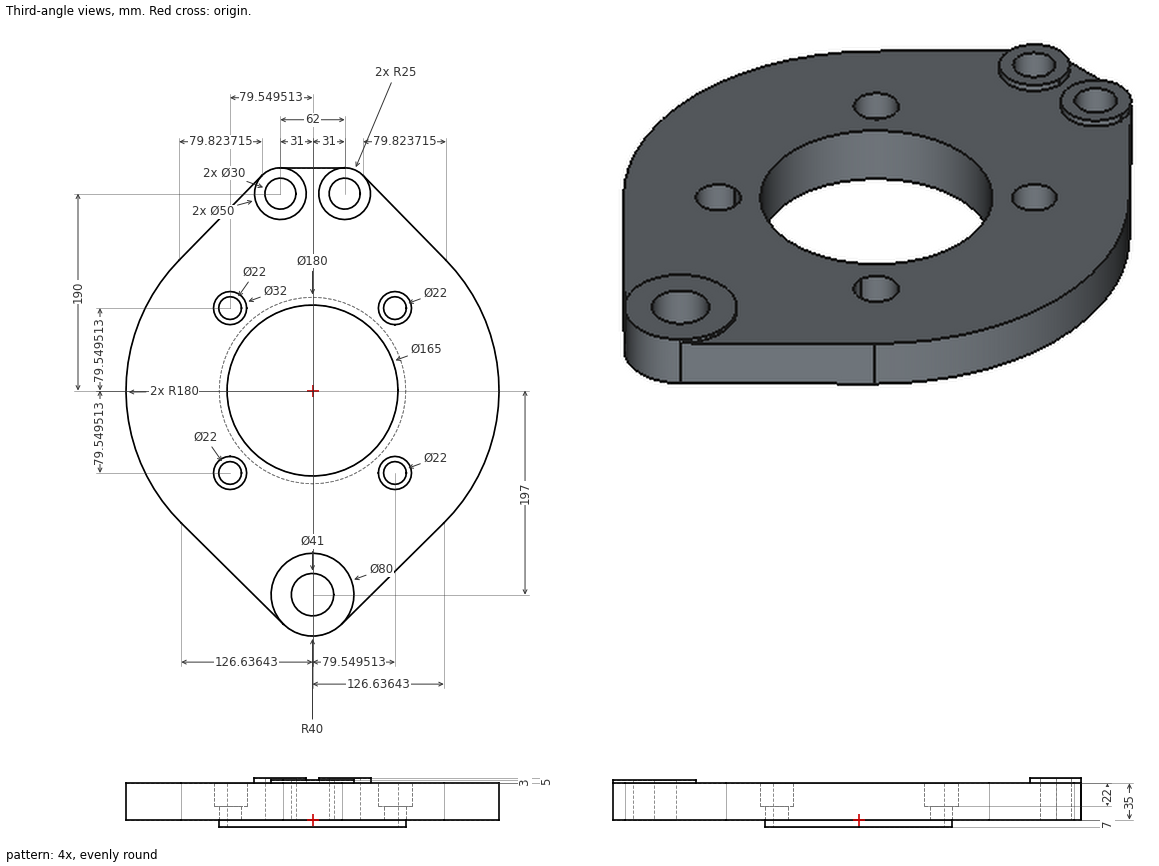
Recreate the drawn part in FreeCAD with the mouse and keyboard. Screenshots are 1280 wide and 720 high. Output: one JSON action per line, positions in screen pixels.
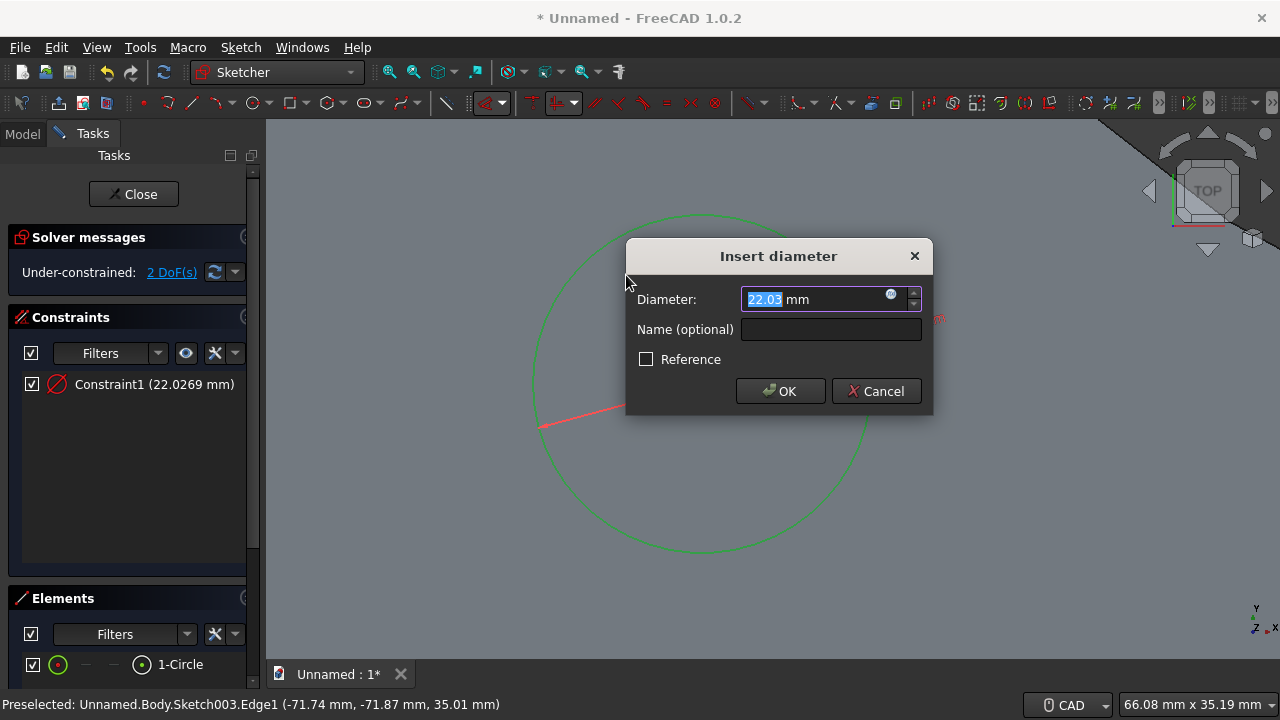
{"action": "type", "text": "22"}
{"action": "key", "text": "Return"}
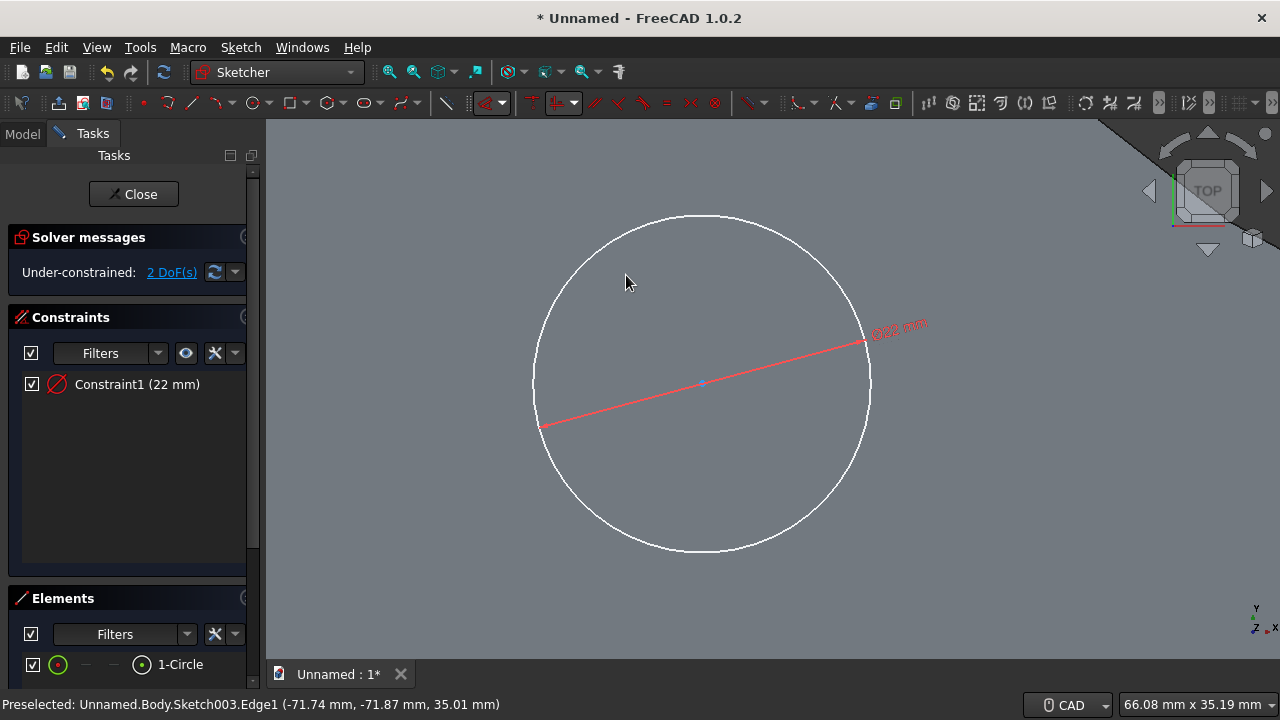
{"action": "left_click", "coordinate": [702, 384]}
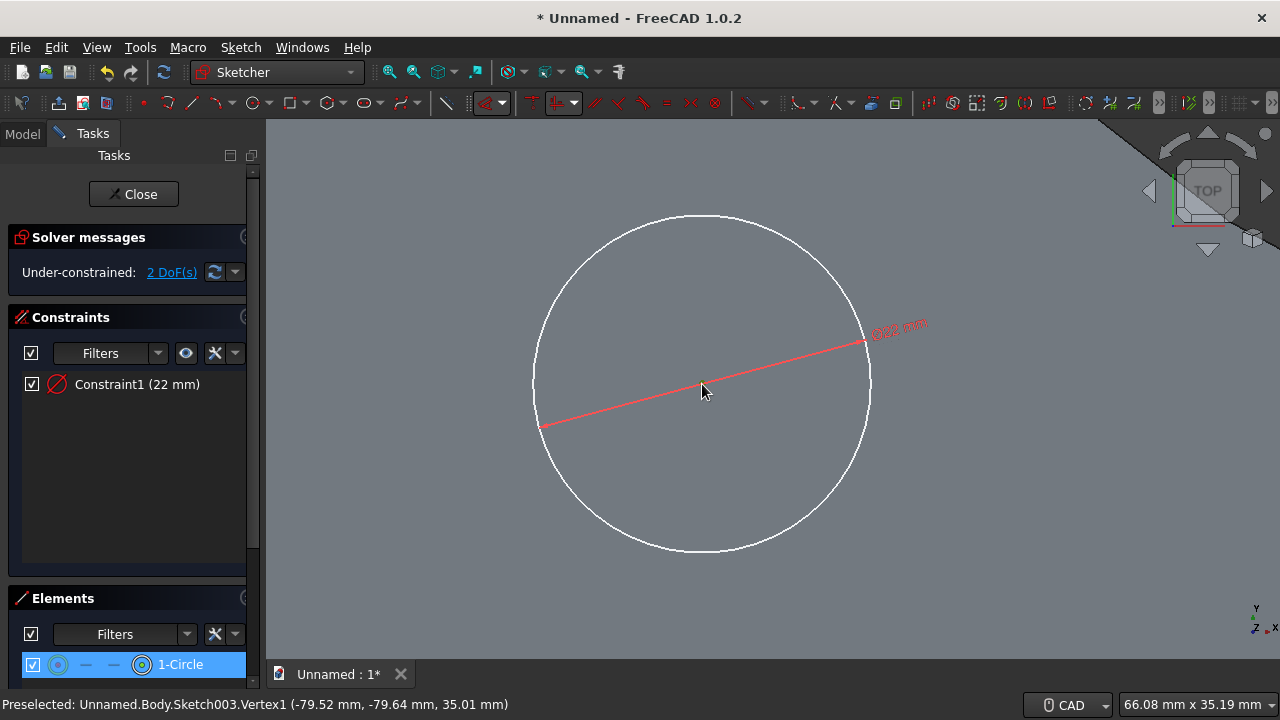
{"action": "key", "text": "l"}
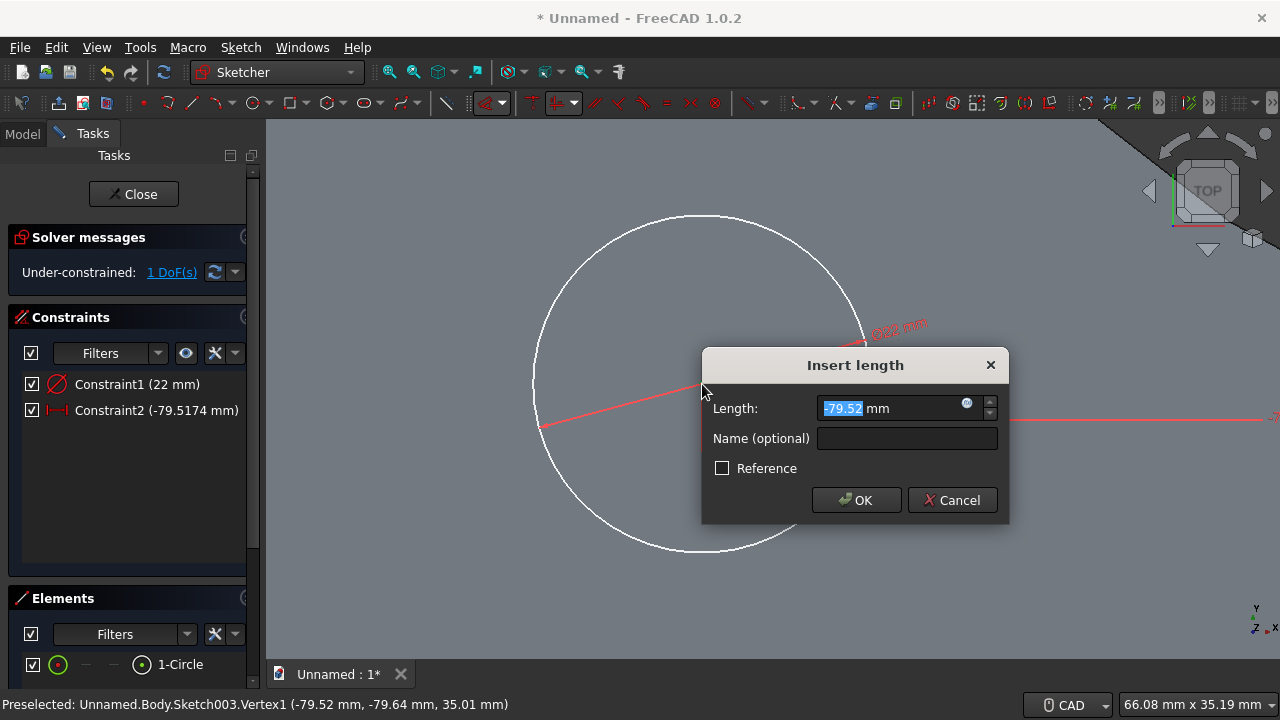
{"action": "type", "text": "-79.549513"}
{"action": "key", "text": "Return"}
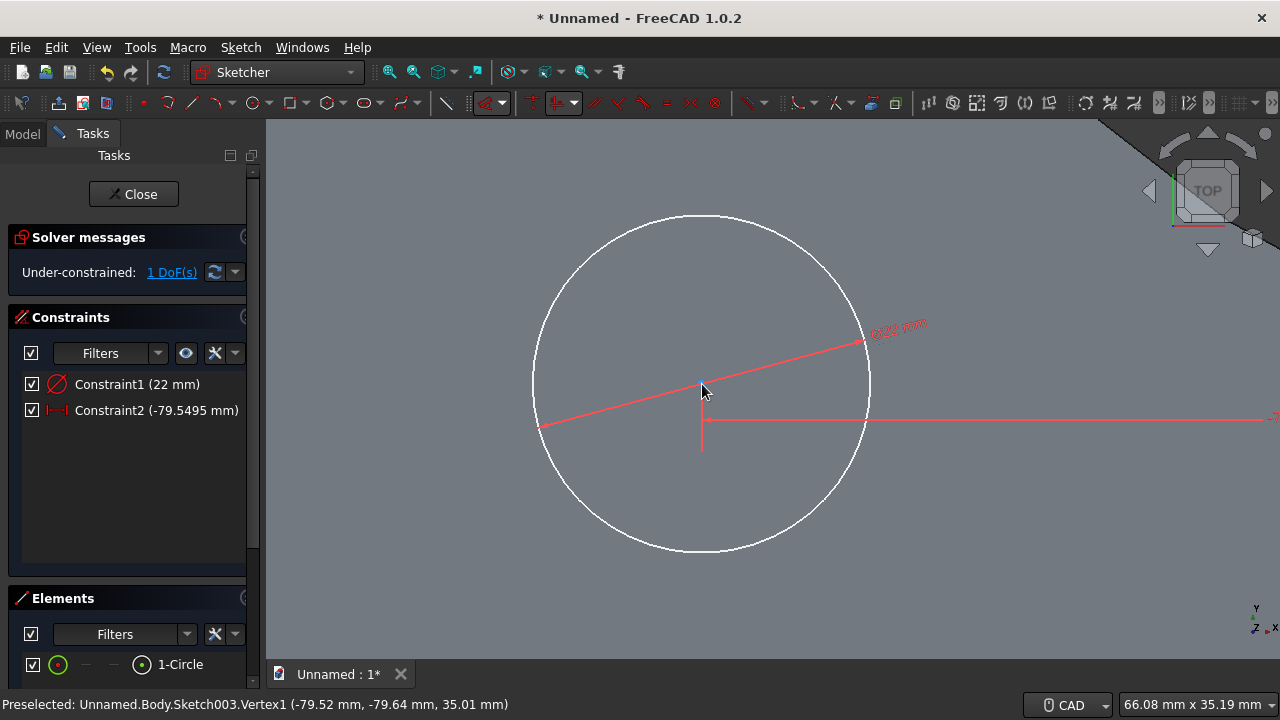
{"action": "left_click", "coordinate": [702, 384]}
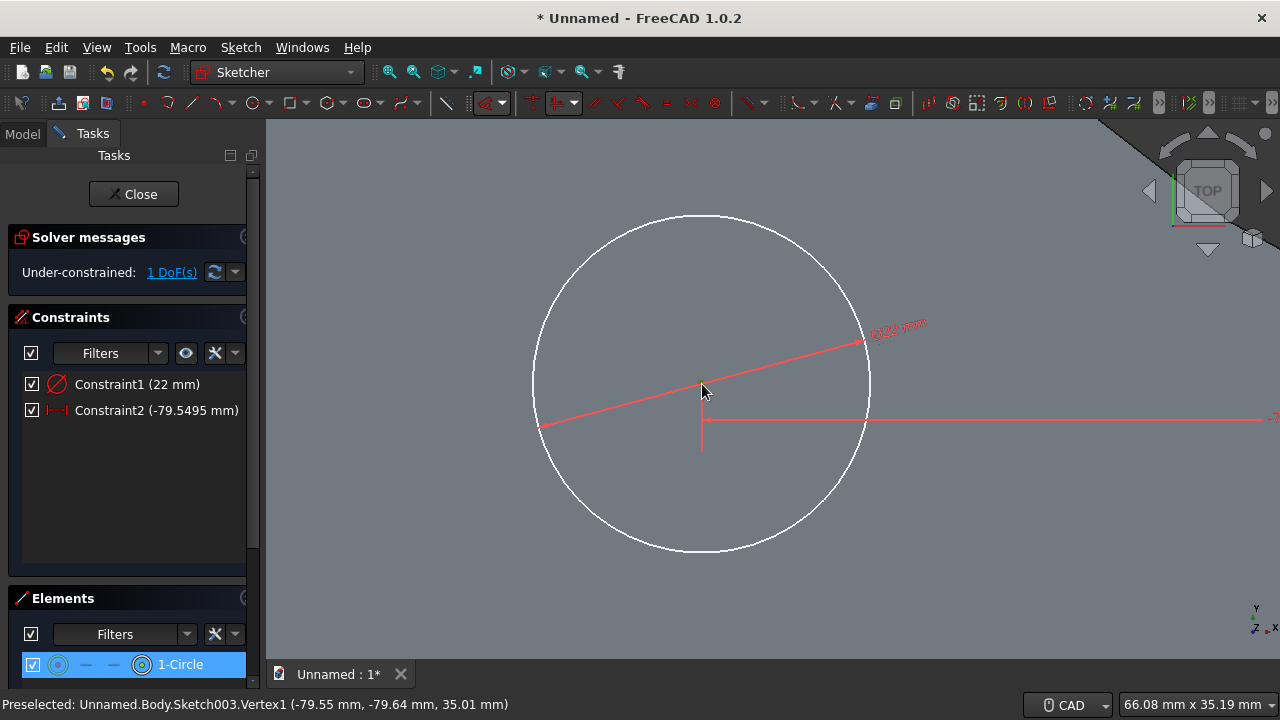
{"action": "left_click", "coordinate": [504, 104]}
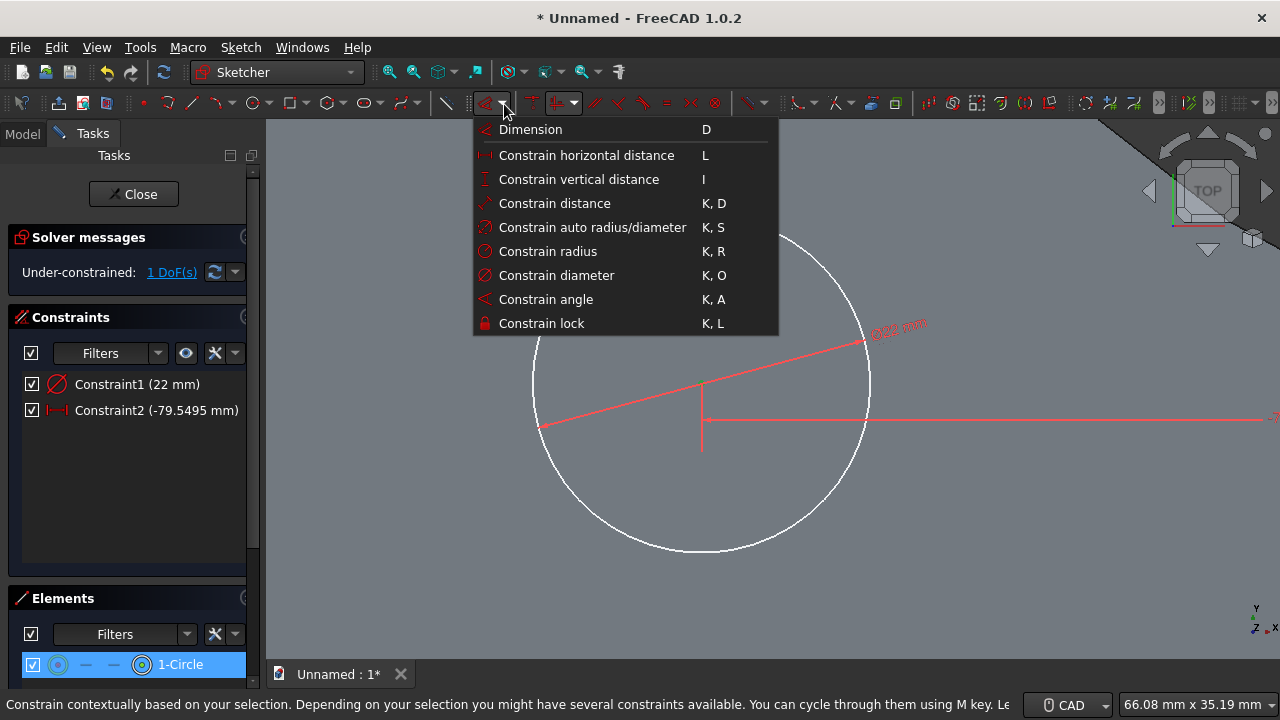
{"action": "left_click", "coordinate": [626, 179]}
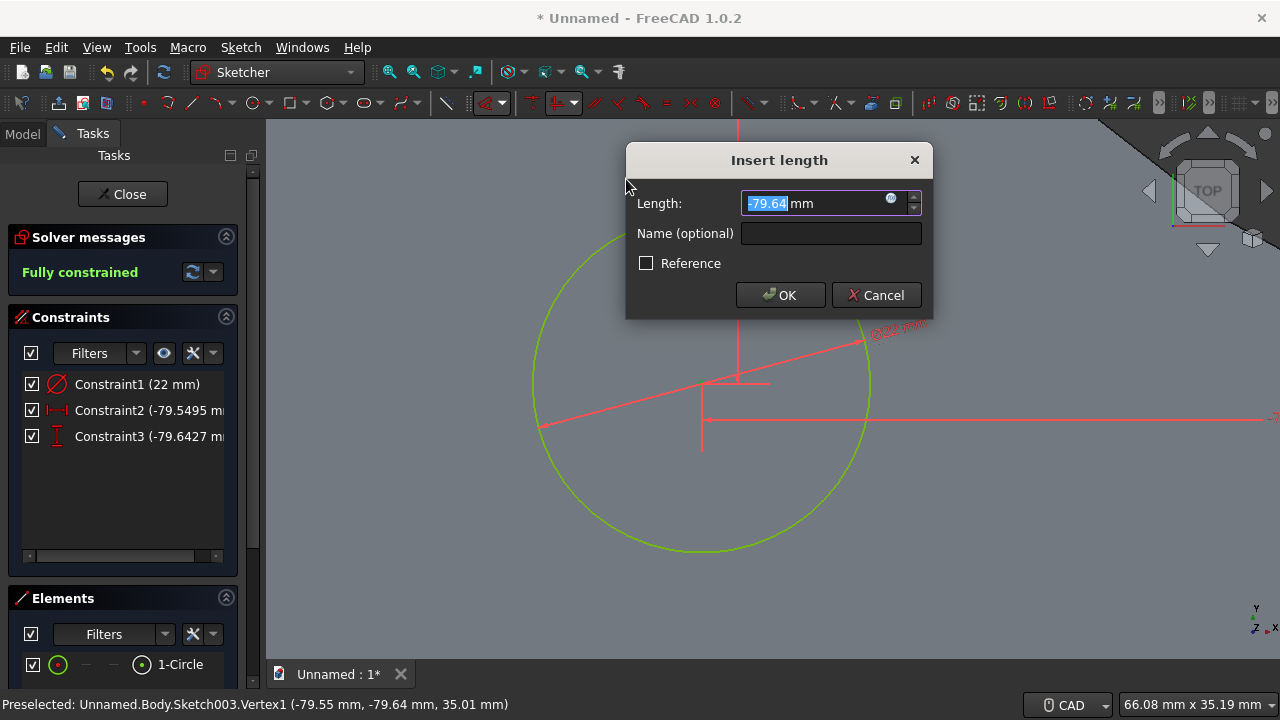
{"action": "type", "text": "-79.549513"}
{"action": "key", "text": "Return"}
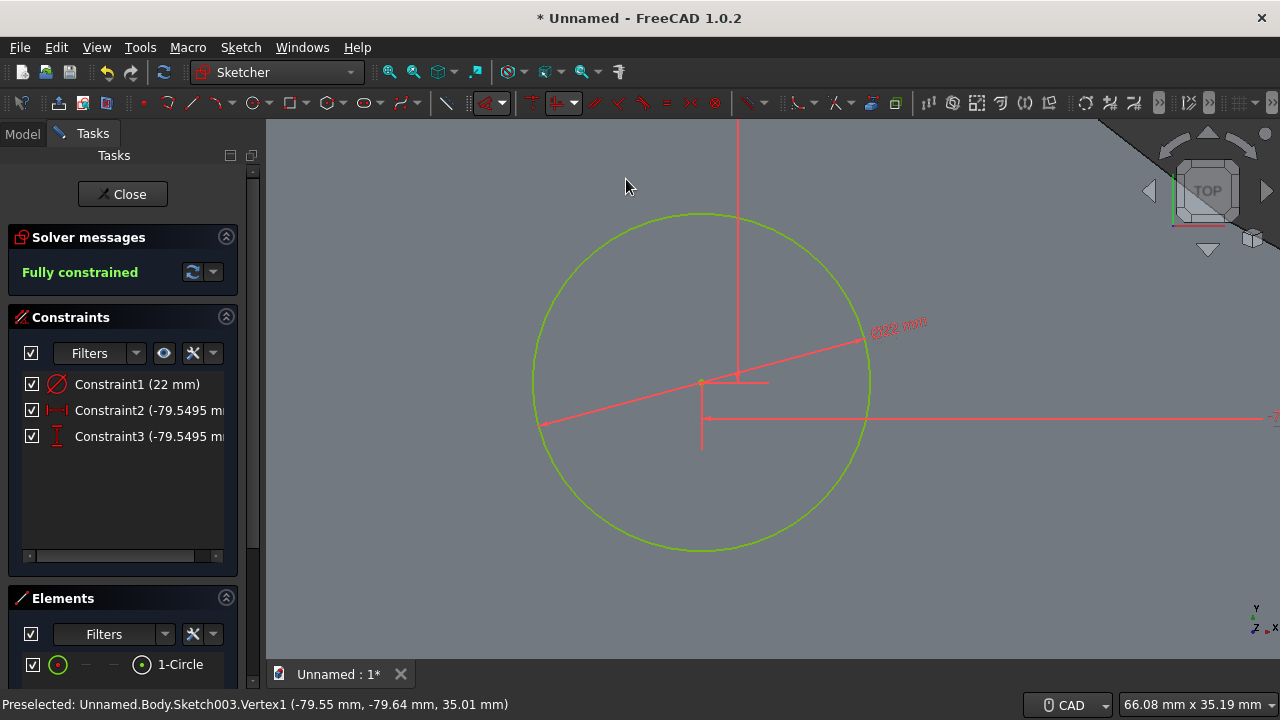
{"action": "left_click", "coordinate": [123, 194]}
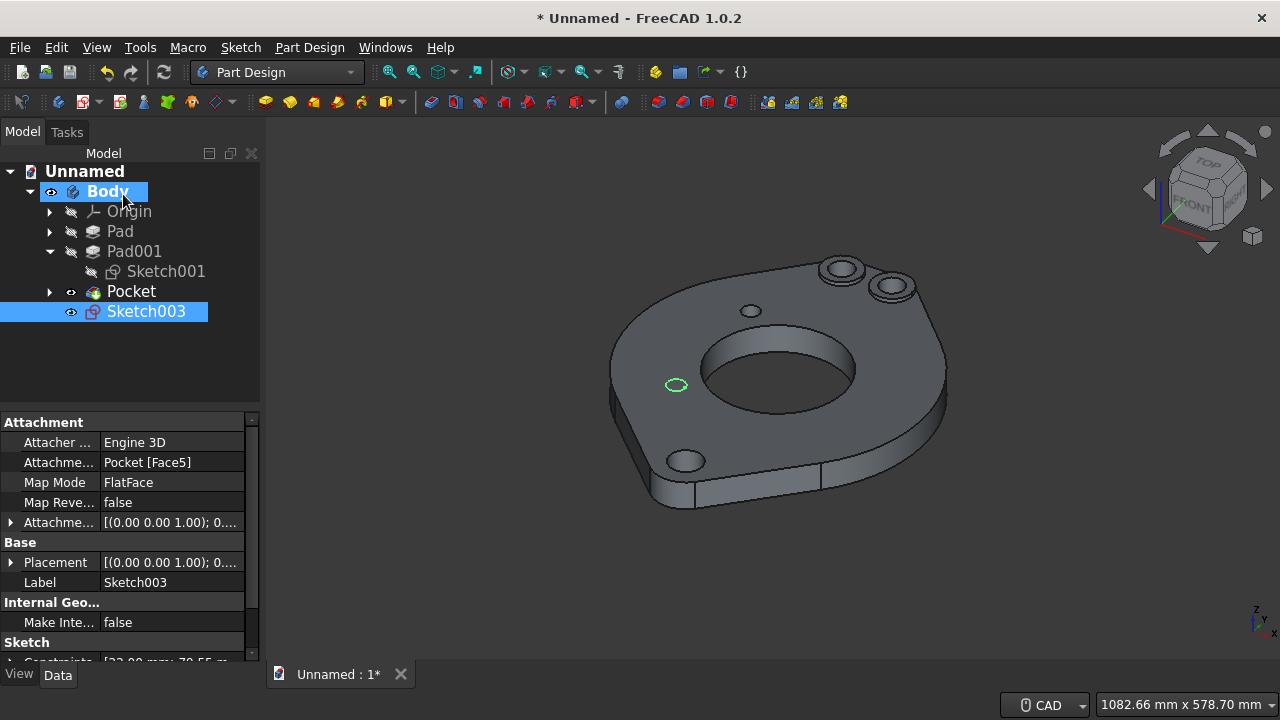
{"action": "left_click", "coordinate": [432, 102]}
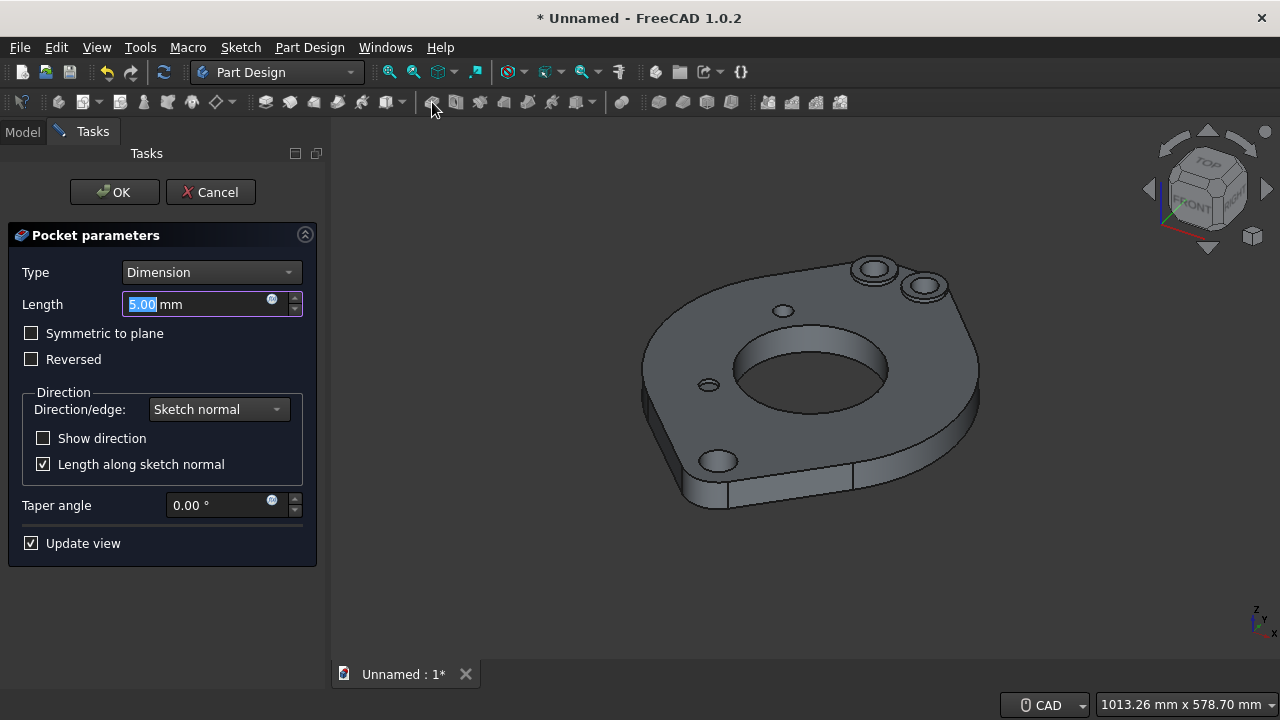
{"action": "left_click", "coordinate": [212, 272]}